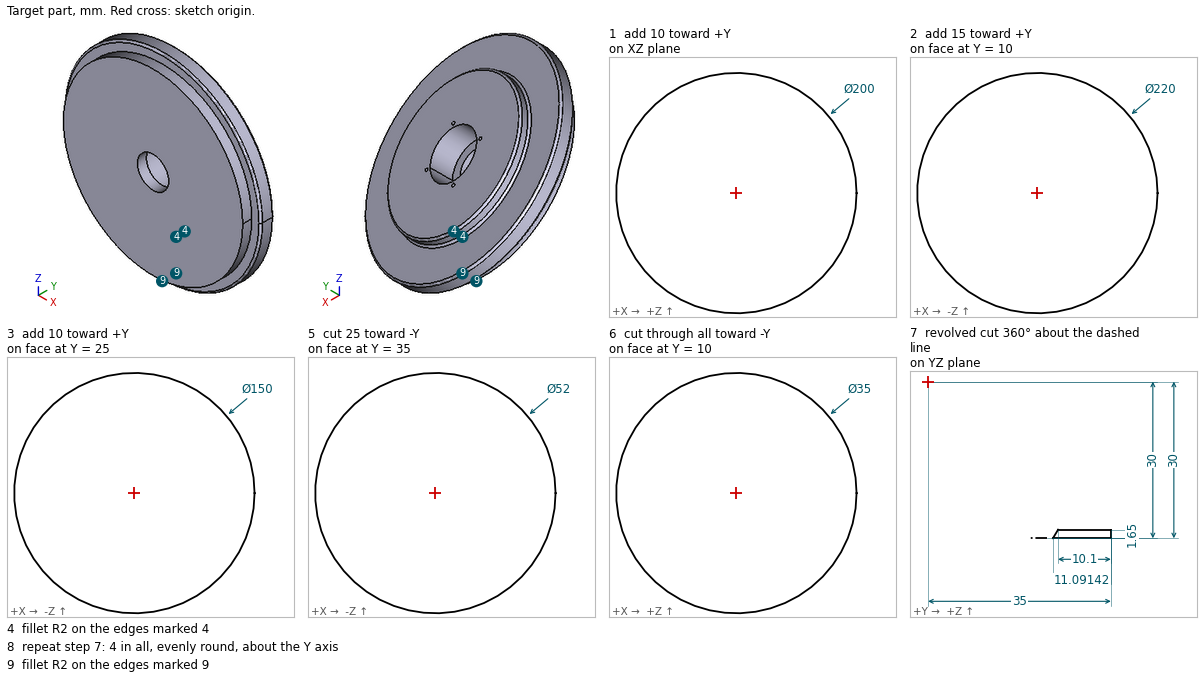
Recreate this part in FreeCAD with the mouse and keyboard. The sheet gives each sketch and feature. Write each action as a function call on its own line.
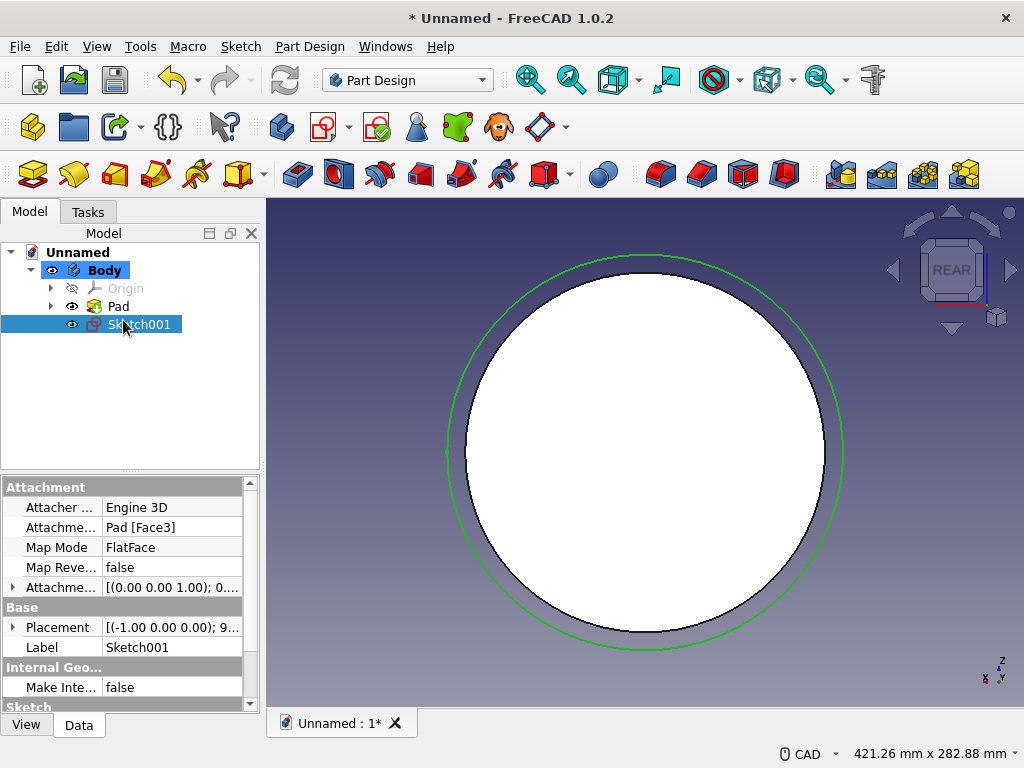
click(33, 174)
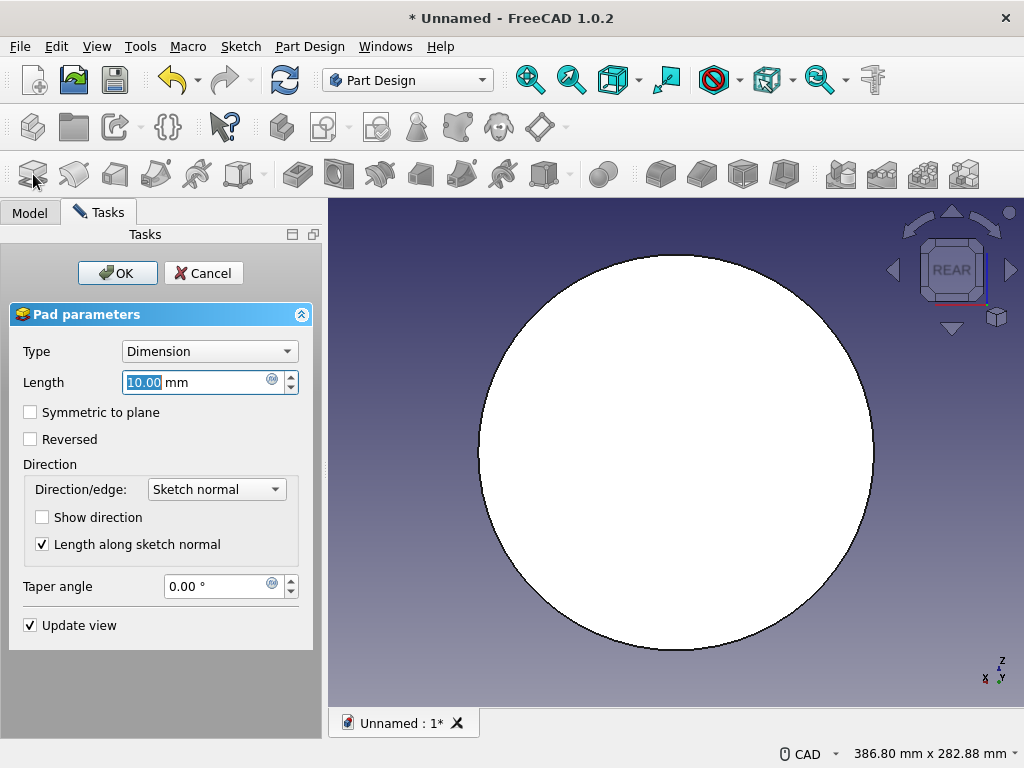
text(15)
key(Tab)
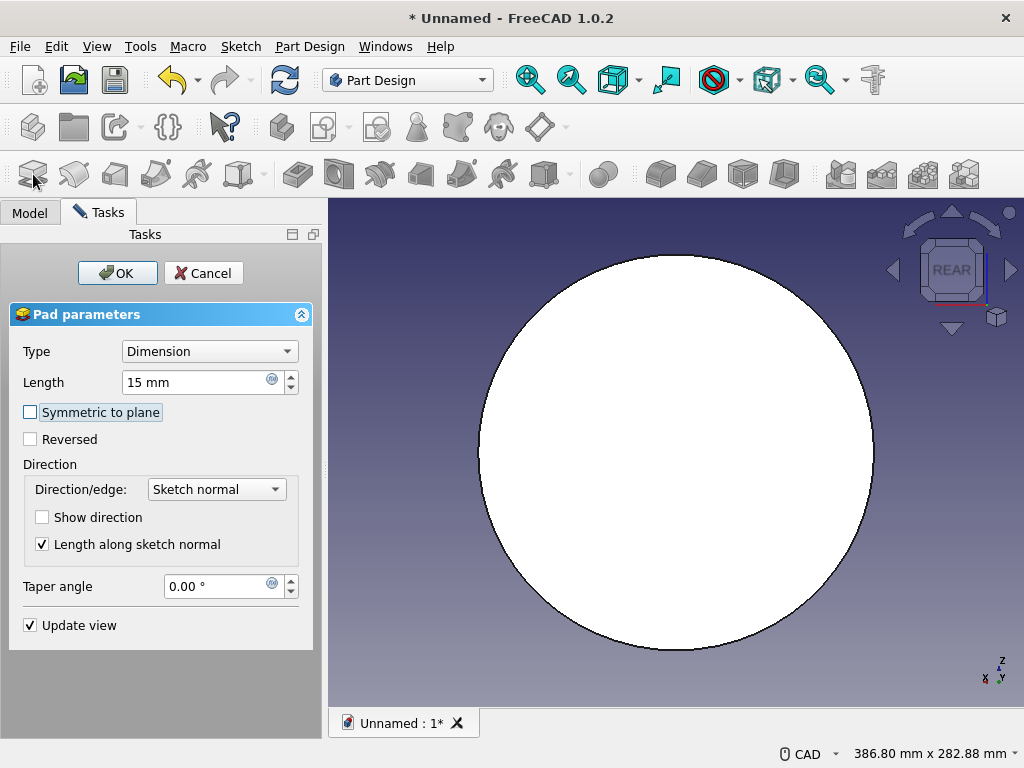
click(118, 273)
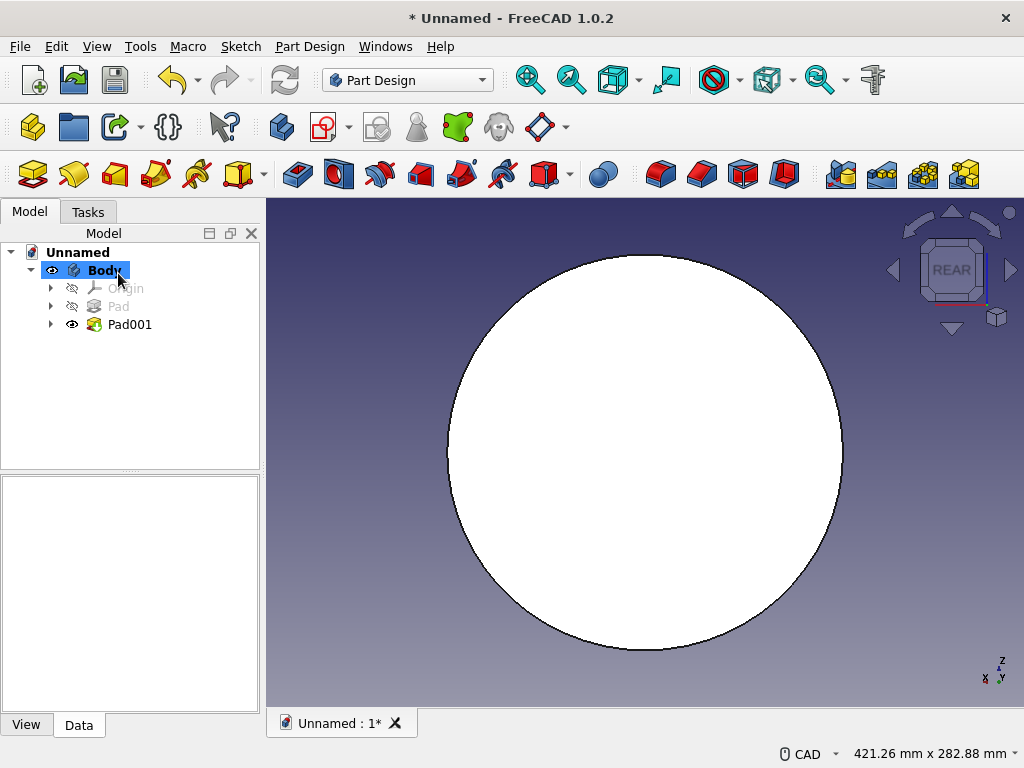
click(645, 451)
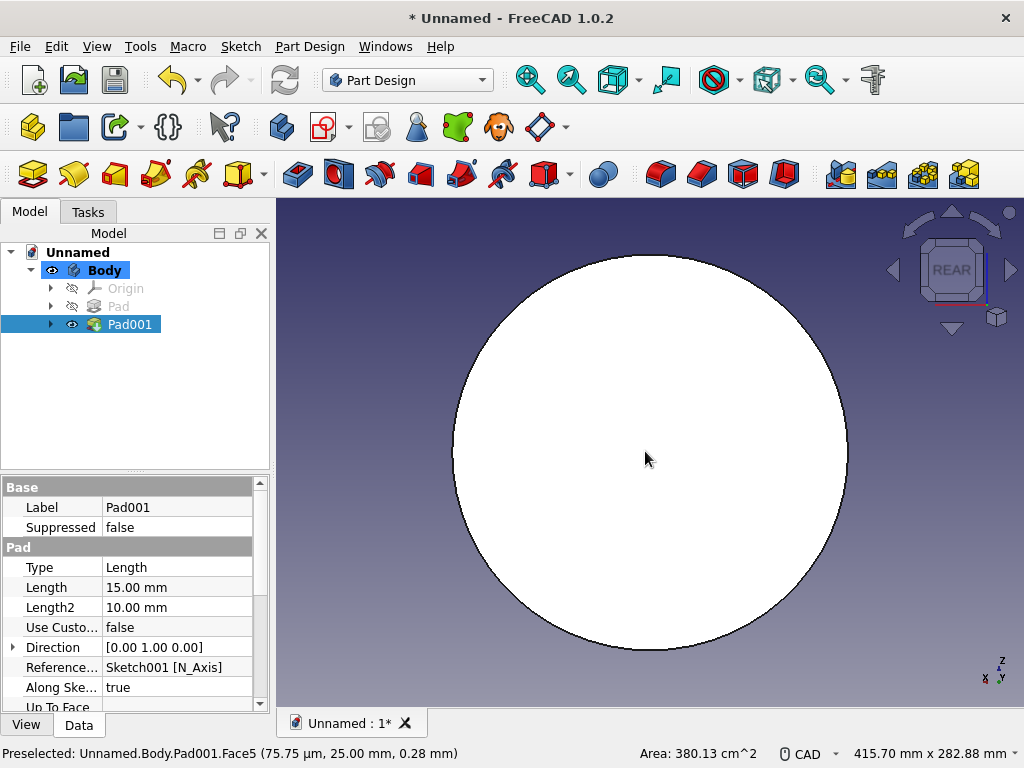
click(322, 128)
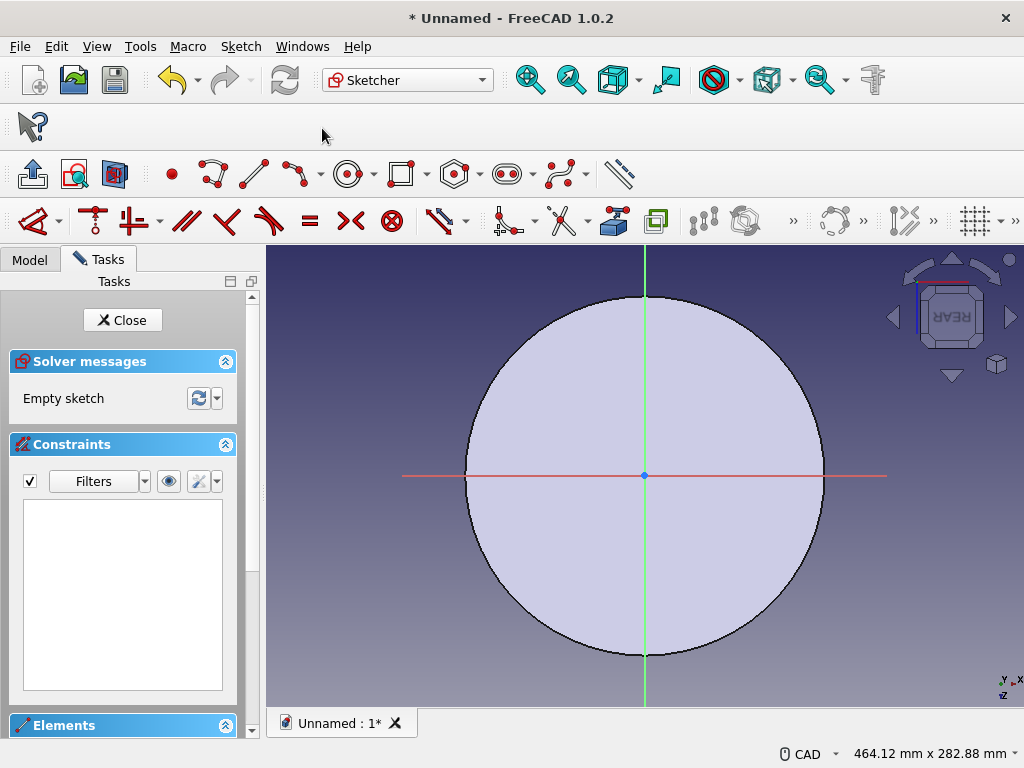
click(348, 174)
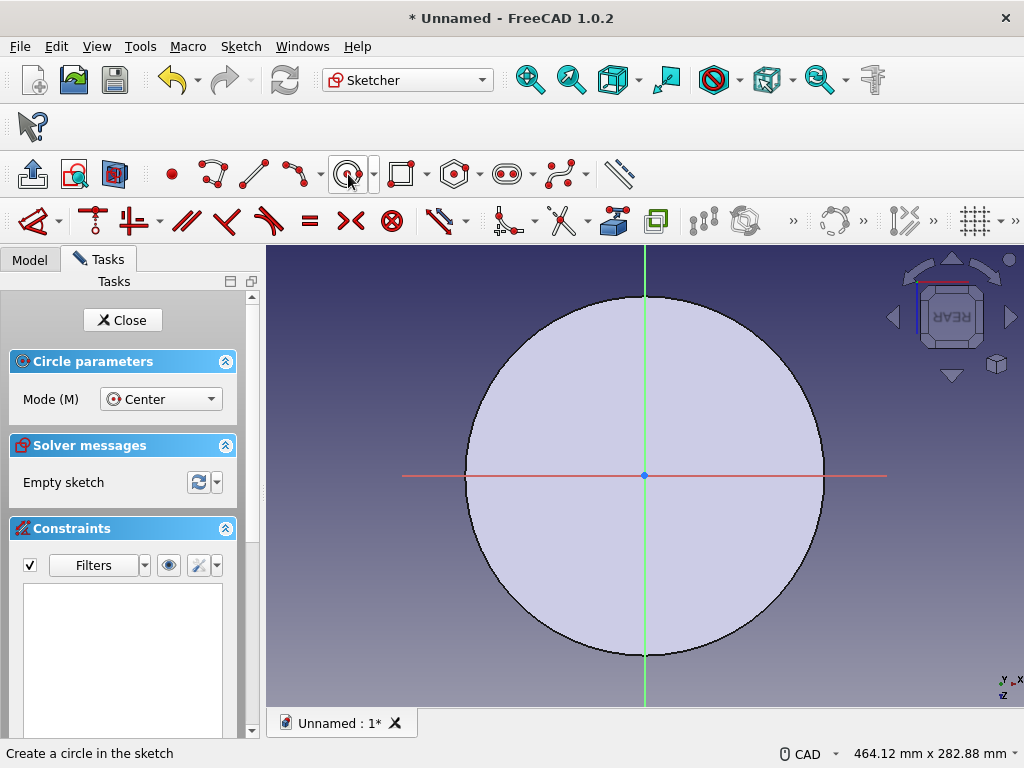
click(645, 476)
click(731, 389)
key(Escape)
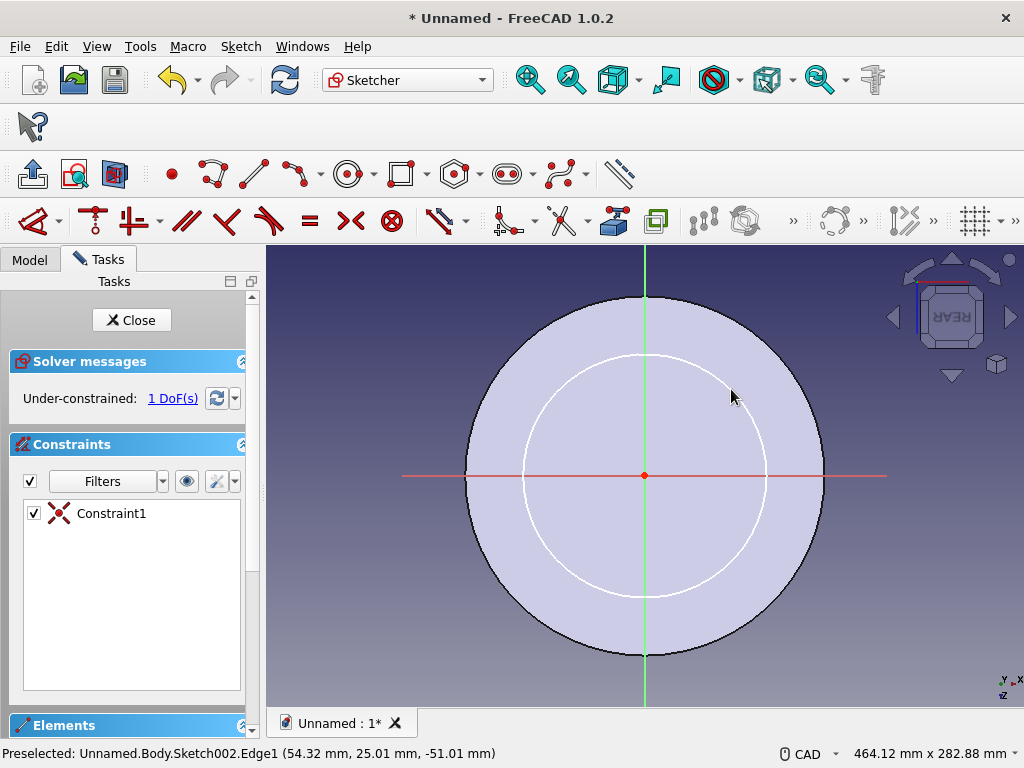
click(32, 222)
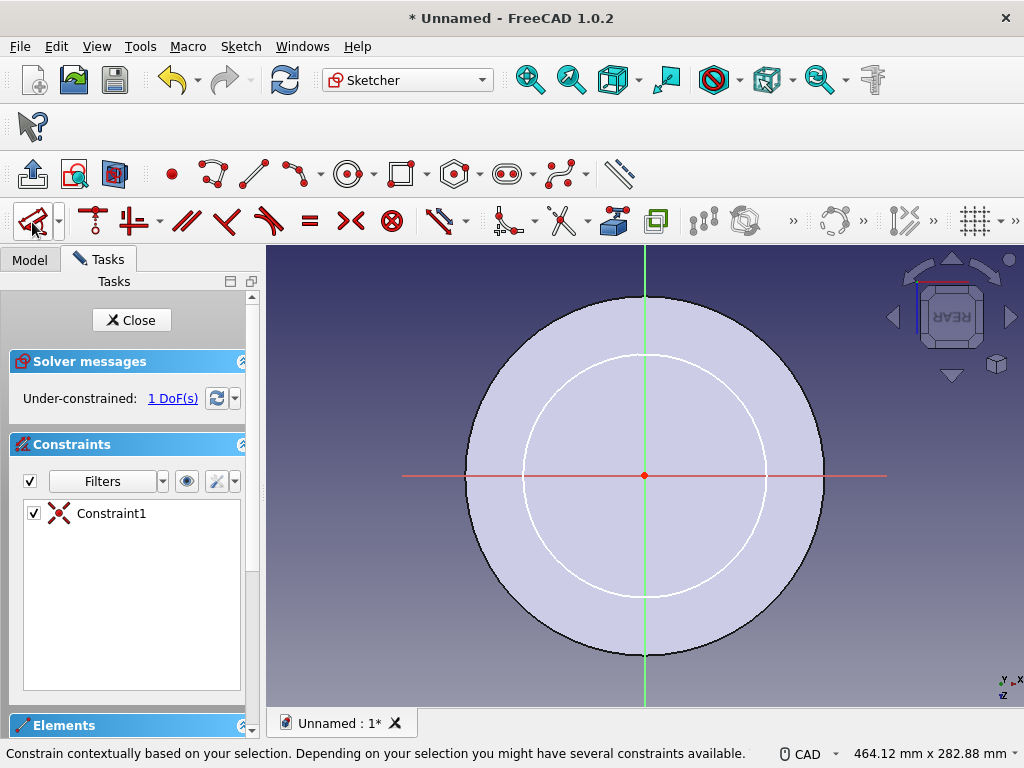
click(731, 390)
click(754, 367)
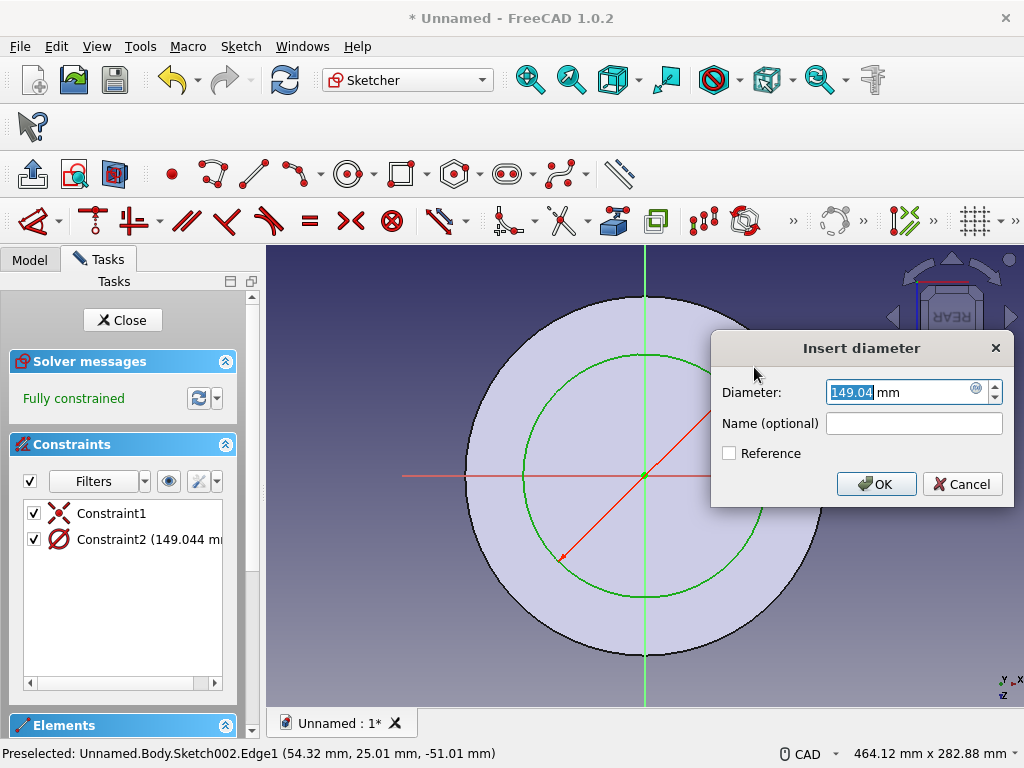
text(150)
key(Return)
key(Escape)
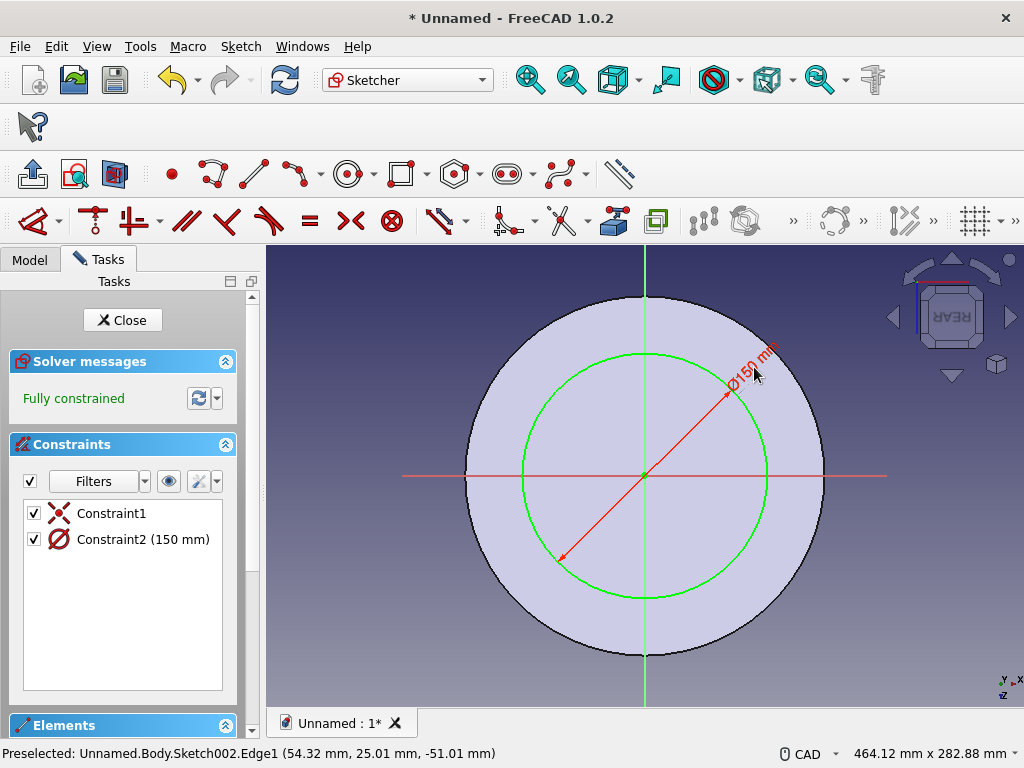
click(123, 320)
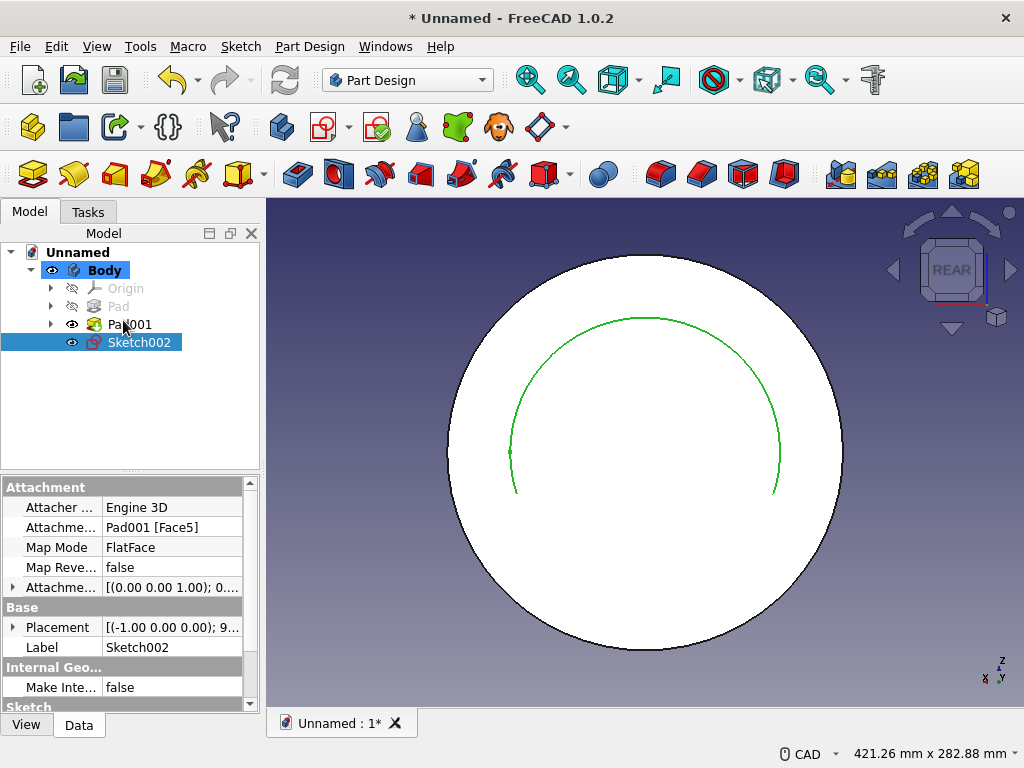
click(33, 174)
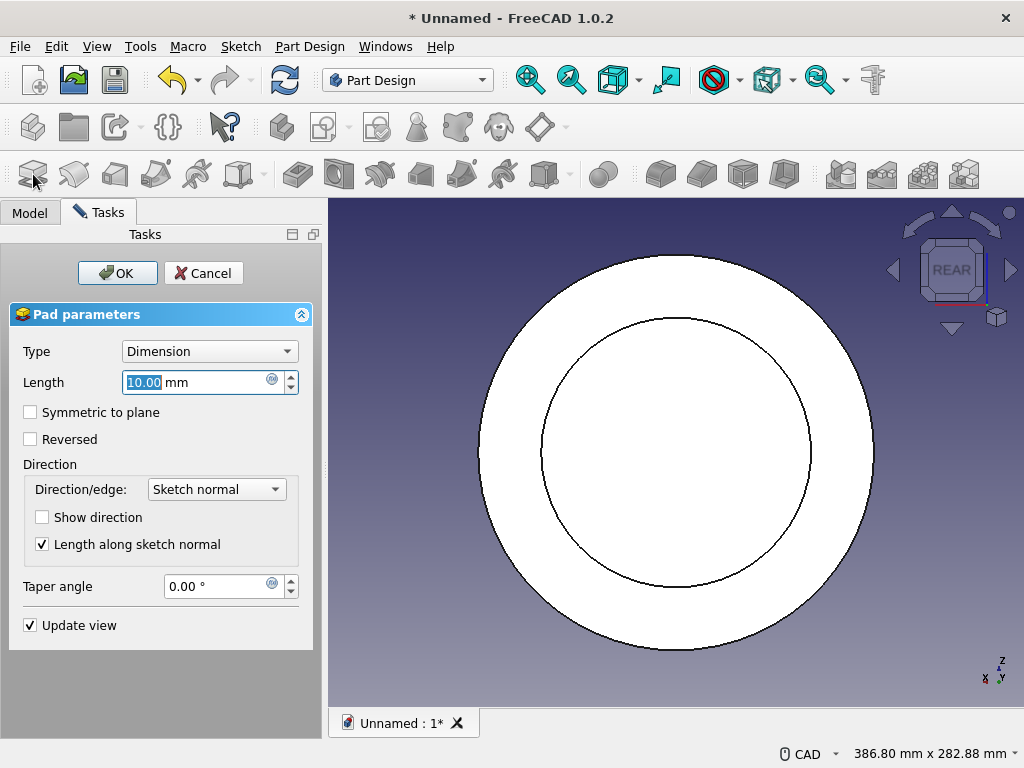
text(10)
key(Tab)